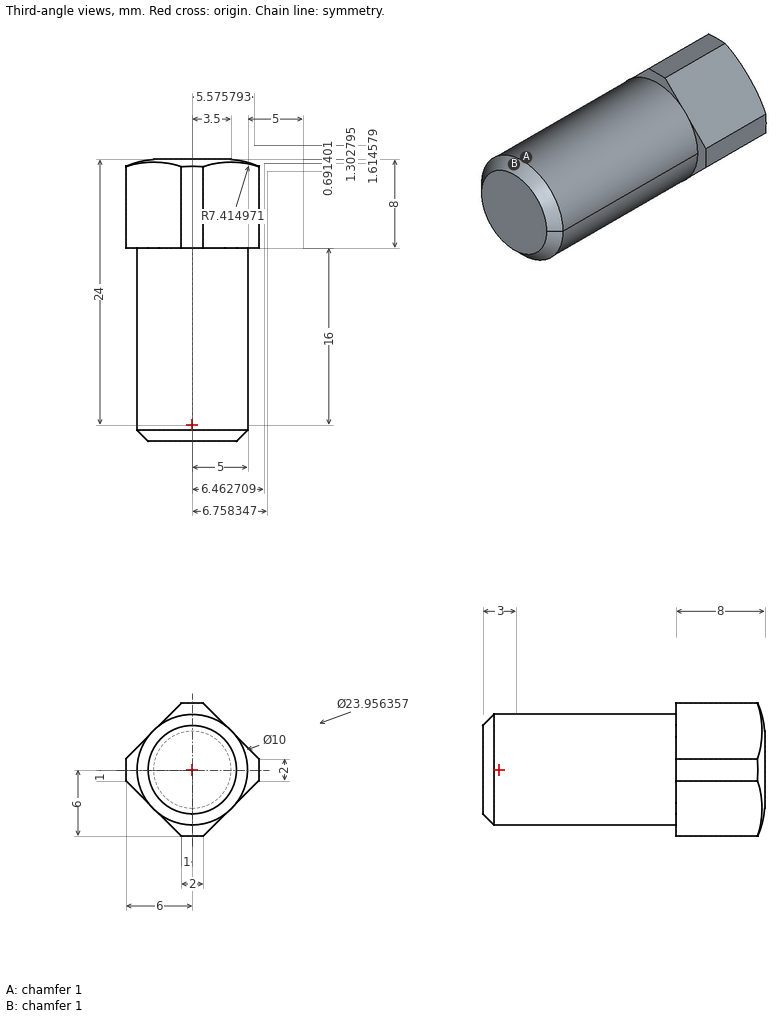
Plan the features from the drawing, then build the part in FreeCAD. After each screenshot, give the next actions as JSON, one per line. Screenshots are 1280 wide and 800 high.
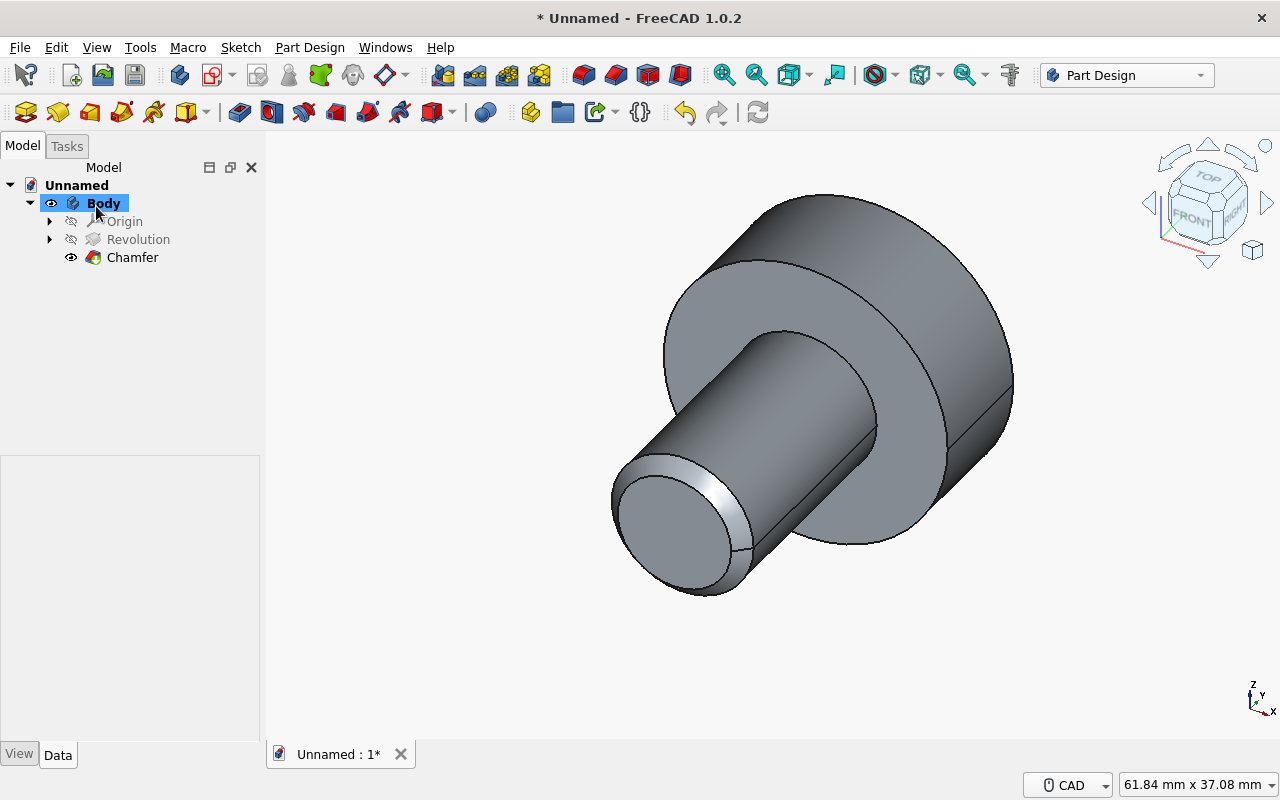
{"action": "key", "text": "4"}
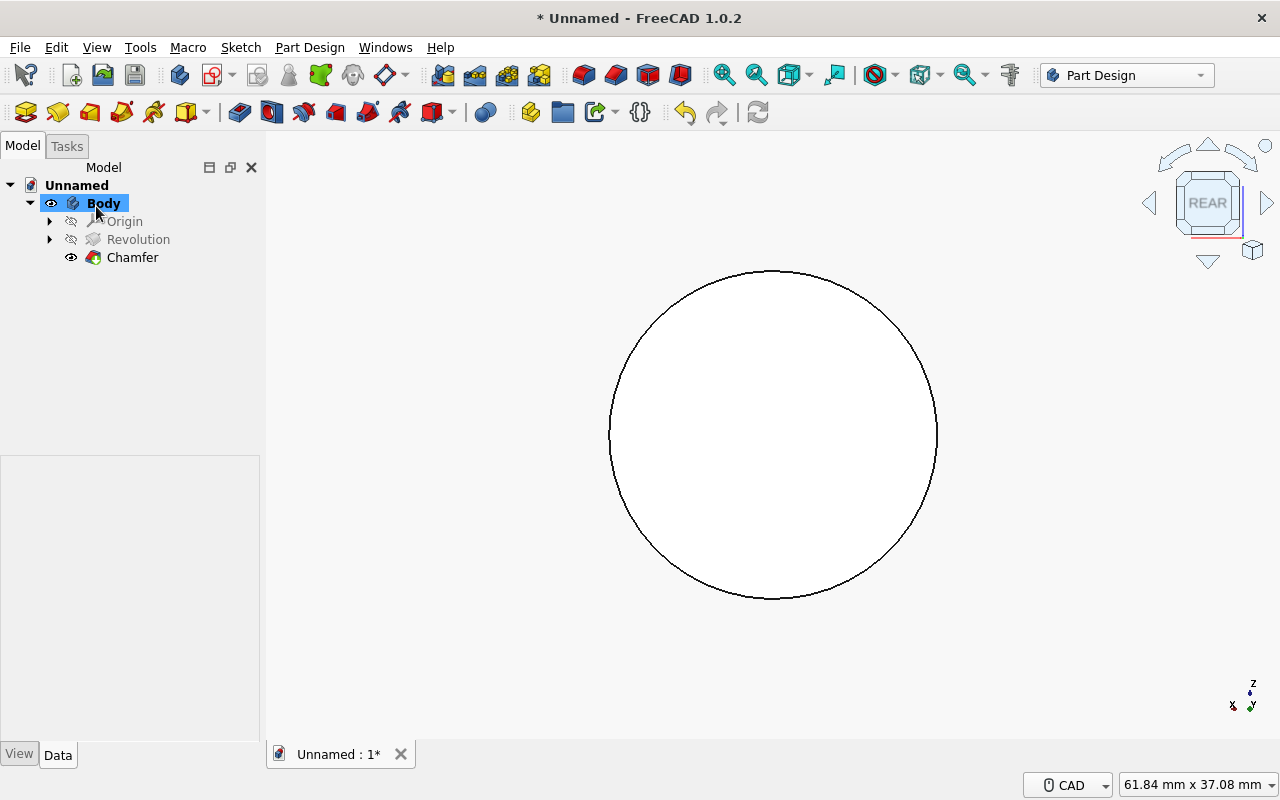
{"action": "left_click", "coordinate": [773, 434]}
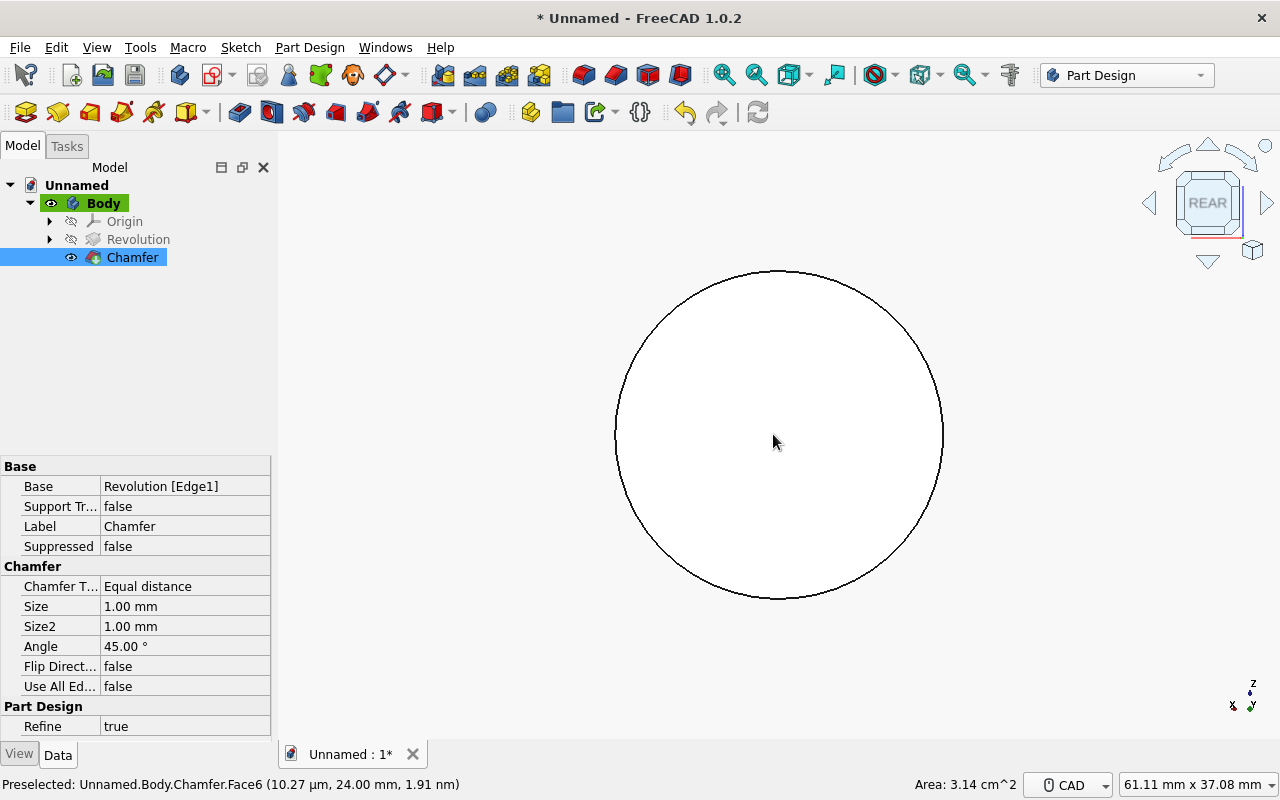
{"action": "left_click", "coordinate": [212, 76]}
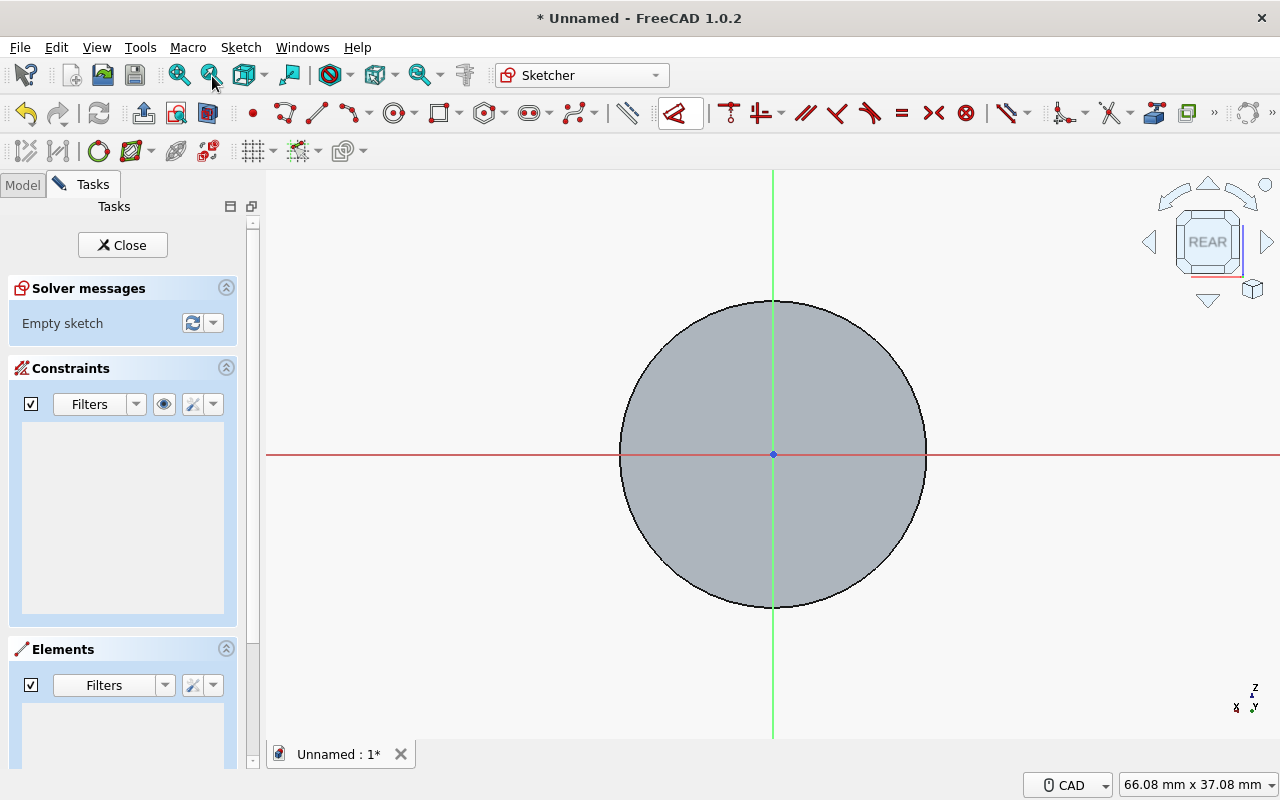
{"action": "key", "text": "g m"}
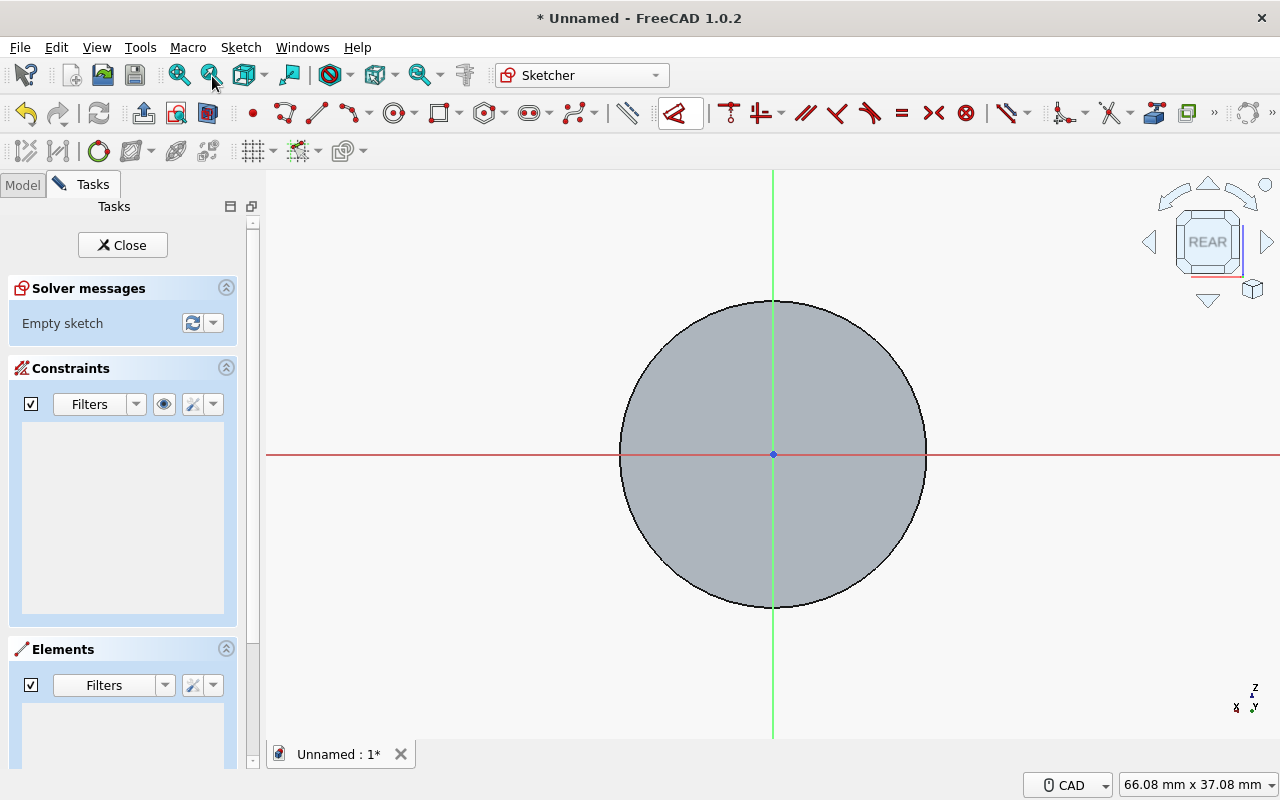
{"action": "left_click", "coordinate": [865, 470]}
{"action": "left_click", "coordinate": [789, 547]}
{"action": "left_click", "coordinate": [758, 547]}
{"action": "left_click", "coordinate": [681, 470]}
{"action": "left_click", "coordinate": [681, 439]}
{"action": "left_click", "coordinate": [758, 362]}
{"action": "left_click", "coordinate": [789, 362]}
{"action": "left_click", "coordinate": [865, 439]}
{"action": "left_click", "coordinate": [865, 471]}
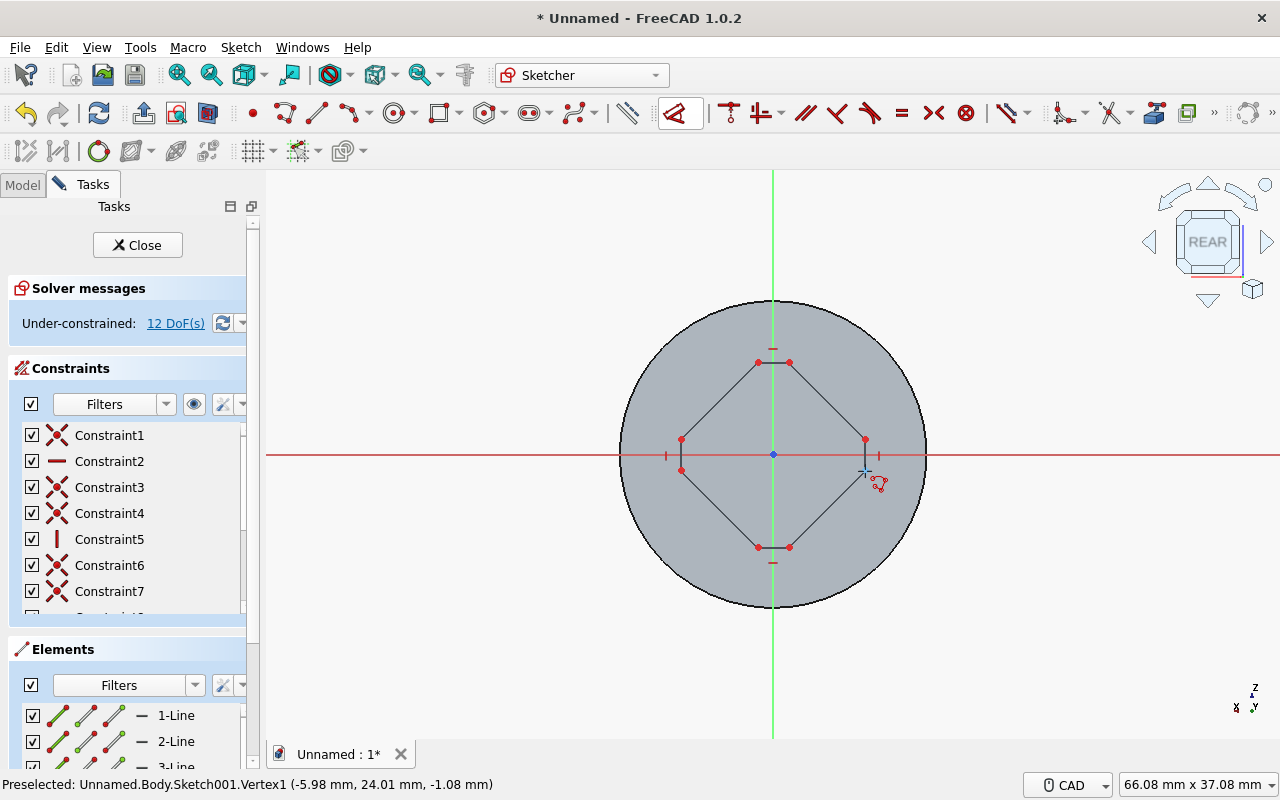
{"action": "left_click", "coordinate": [394, 114]}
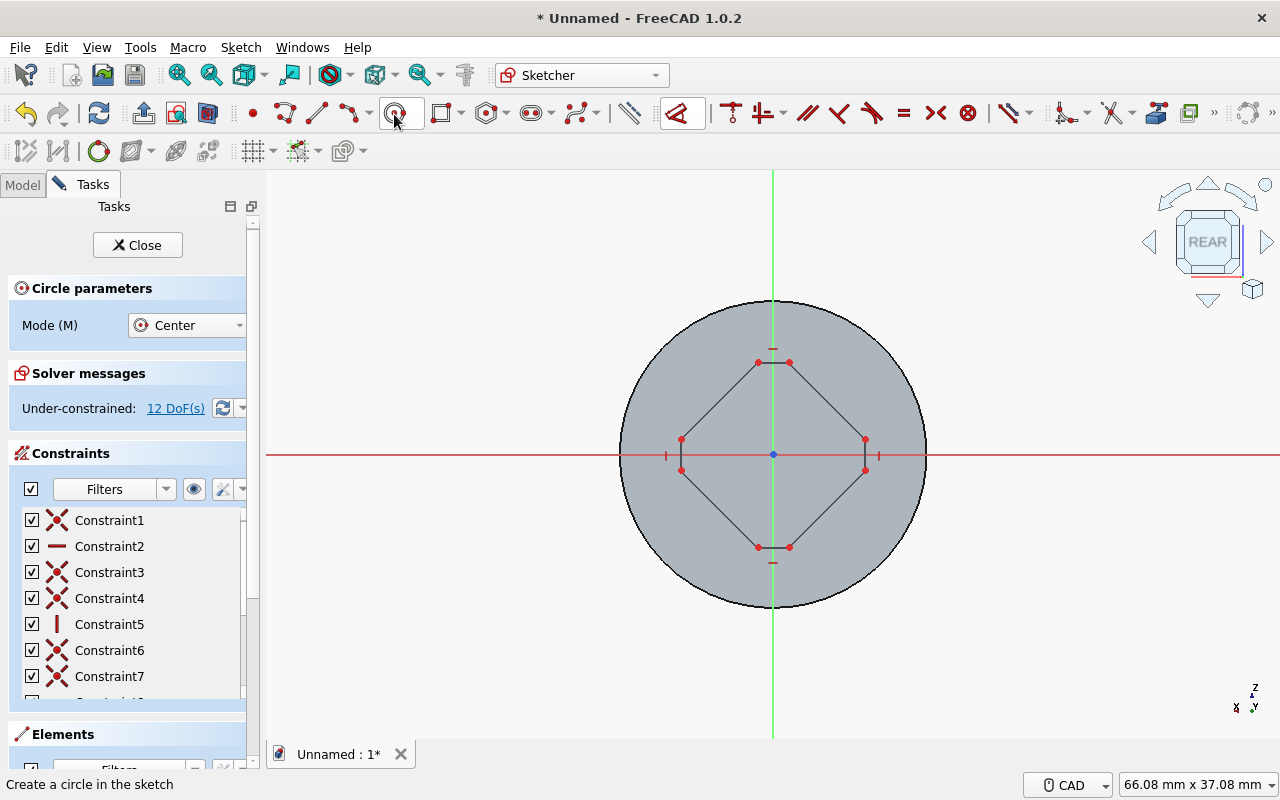
{"action": "left_click", "coordinate": [773, 455]}
{"action": "left_click", "coordinate": [903, 325]}
{"action": "key", "text": "Escape"}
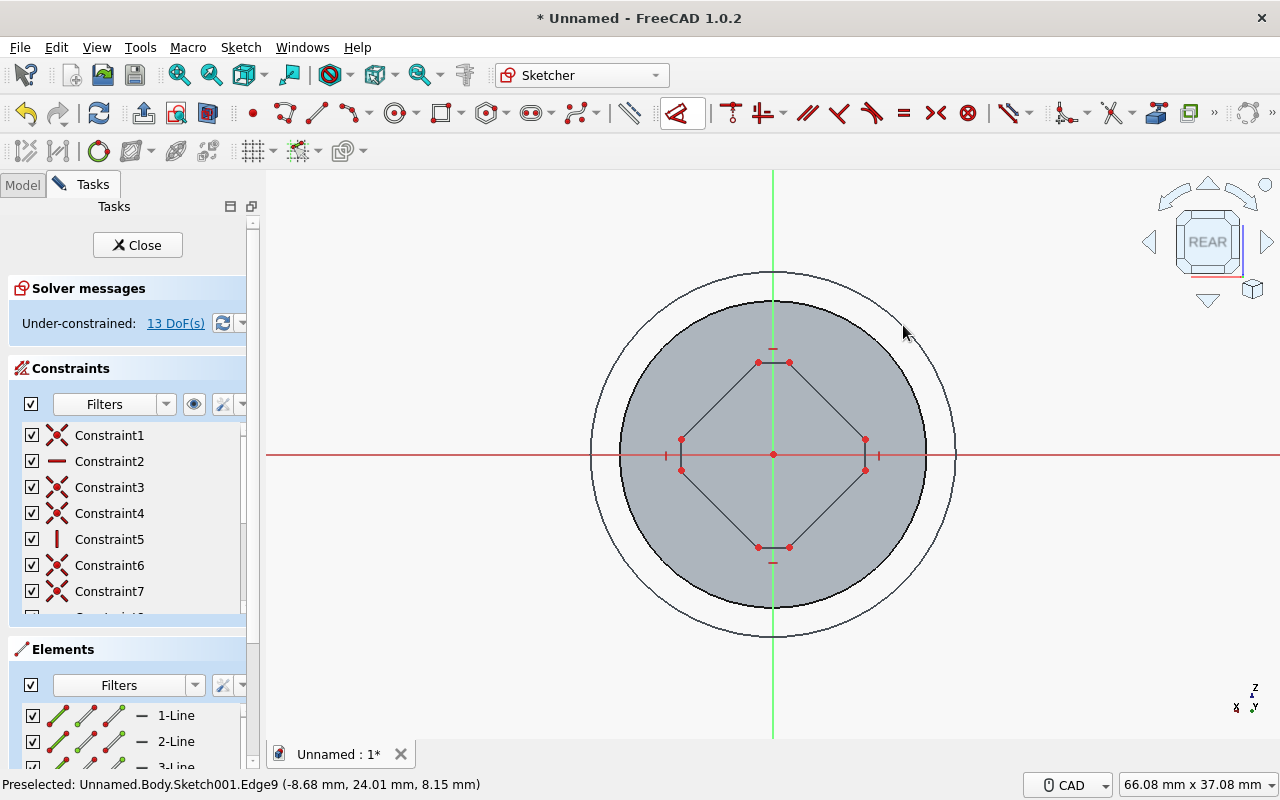
{"action": "left_click", "coordinate": [865, 471]}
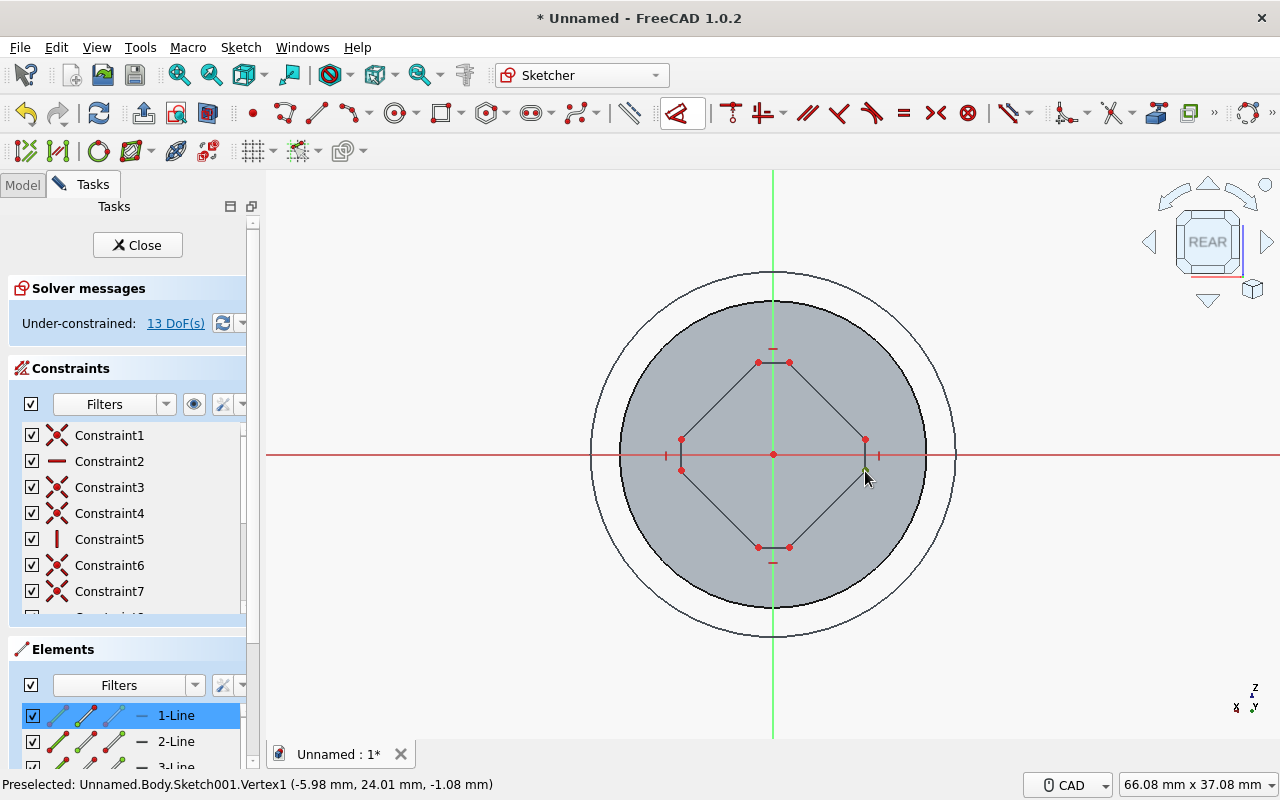
{"action": "left_click", "coordinate": [681, 471]}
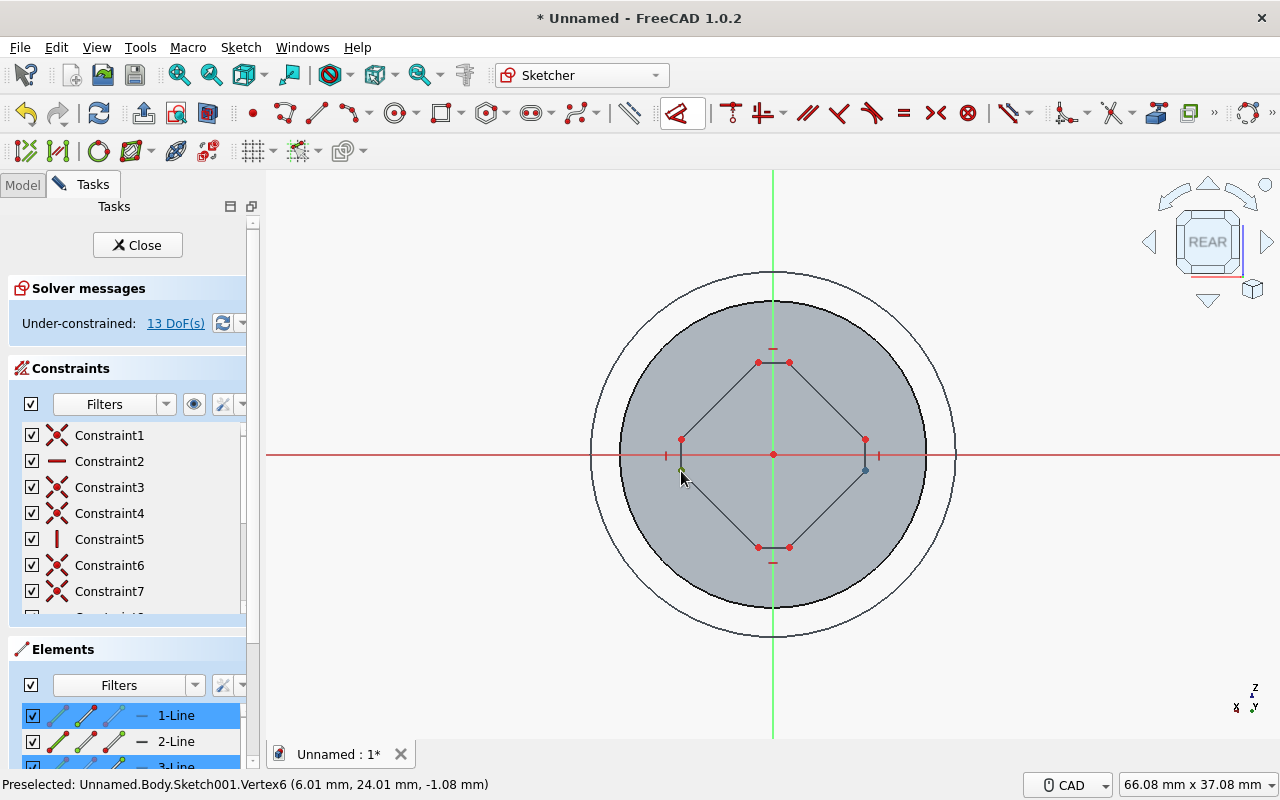
{"action": "left_click", "coordinate": [773, 674]}